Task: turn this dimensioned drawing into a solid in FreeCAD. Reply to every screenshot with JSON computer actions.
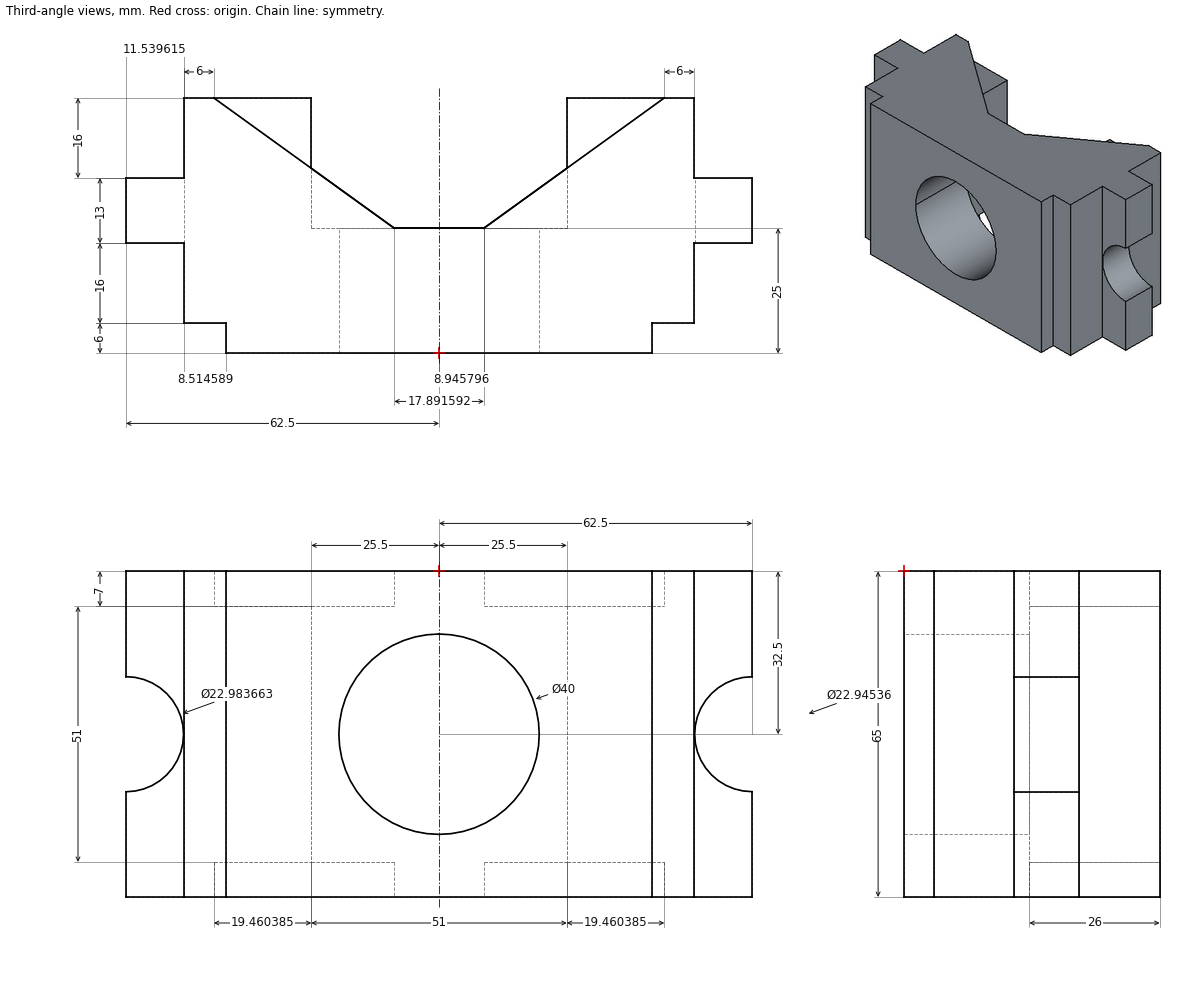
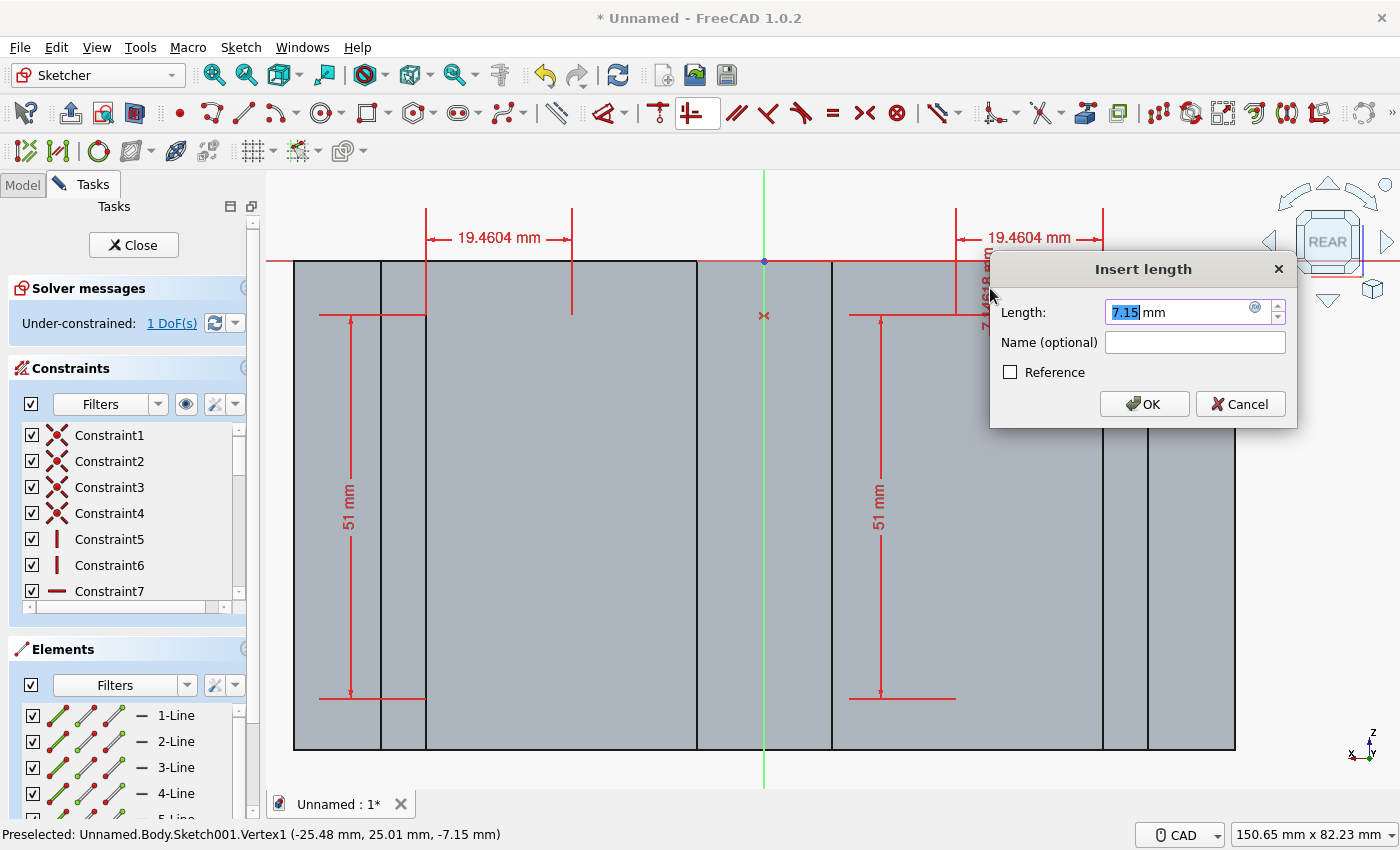
{"action": "type", "text": "7"}
{"action": "key", "text": "Return"}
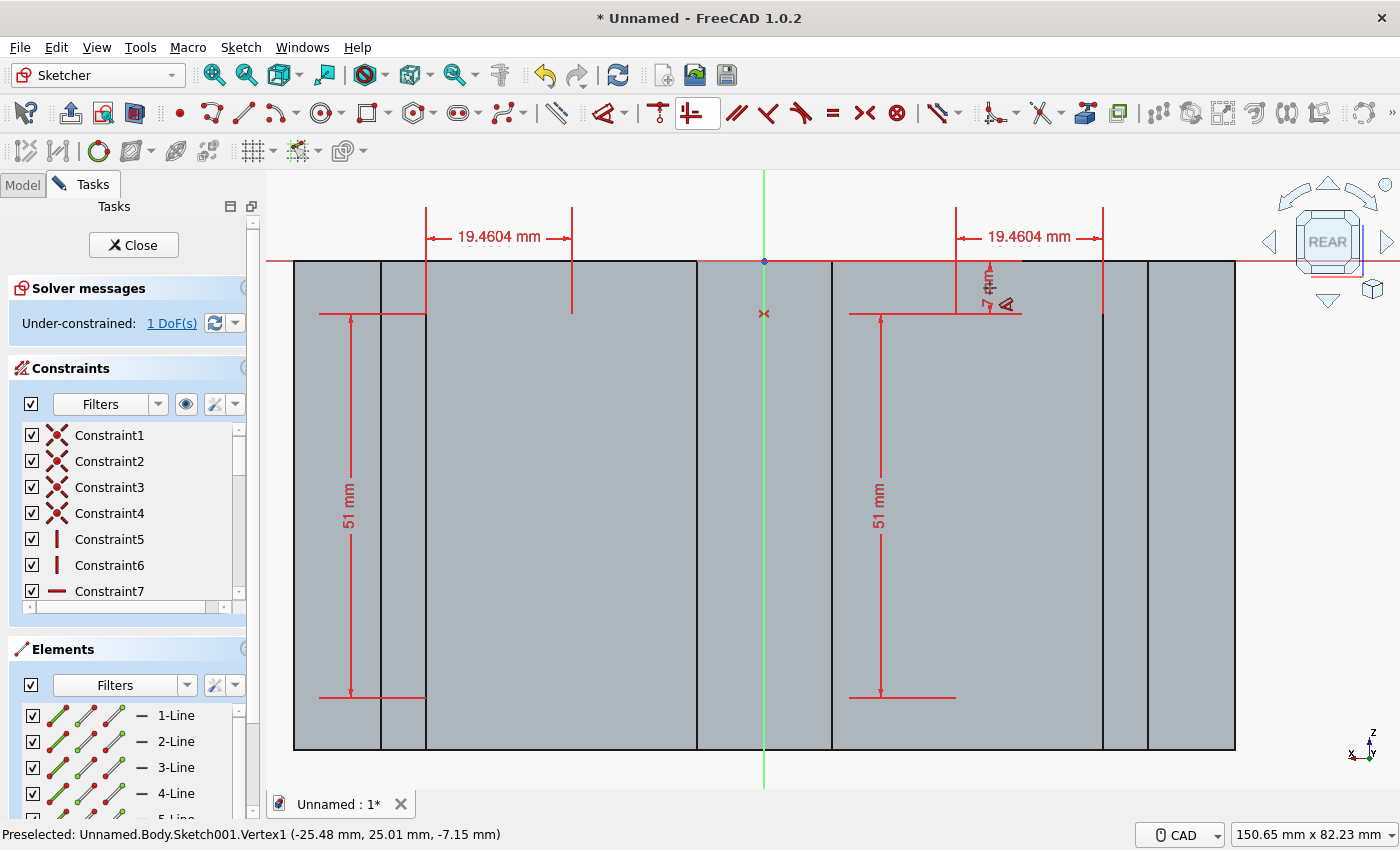
{"action": "left_click", "coordinate": [956, 314]}
{"action": "left_click", "coordinate": [860, 227]}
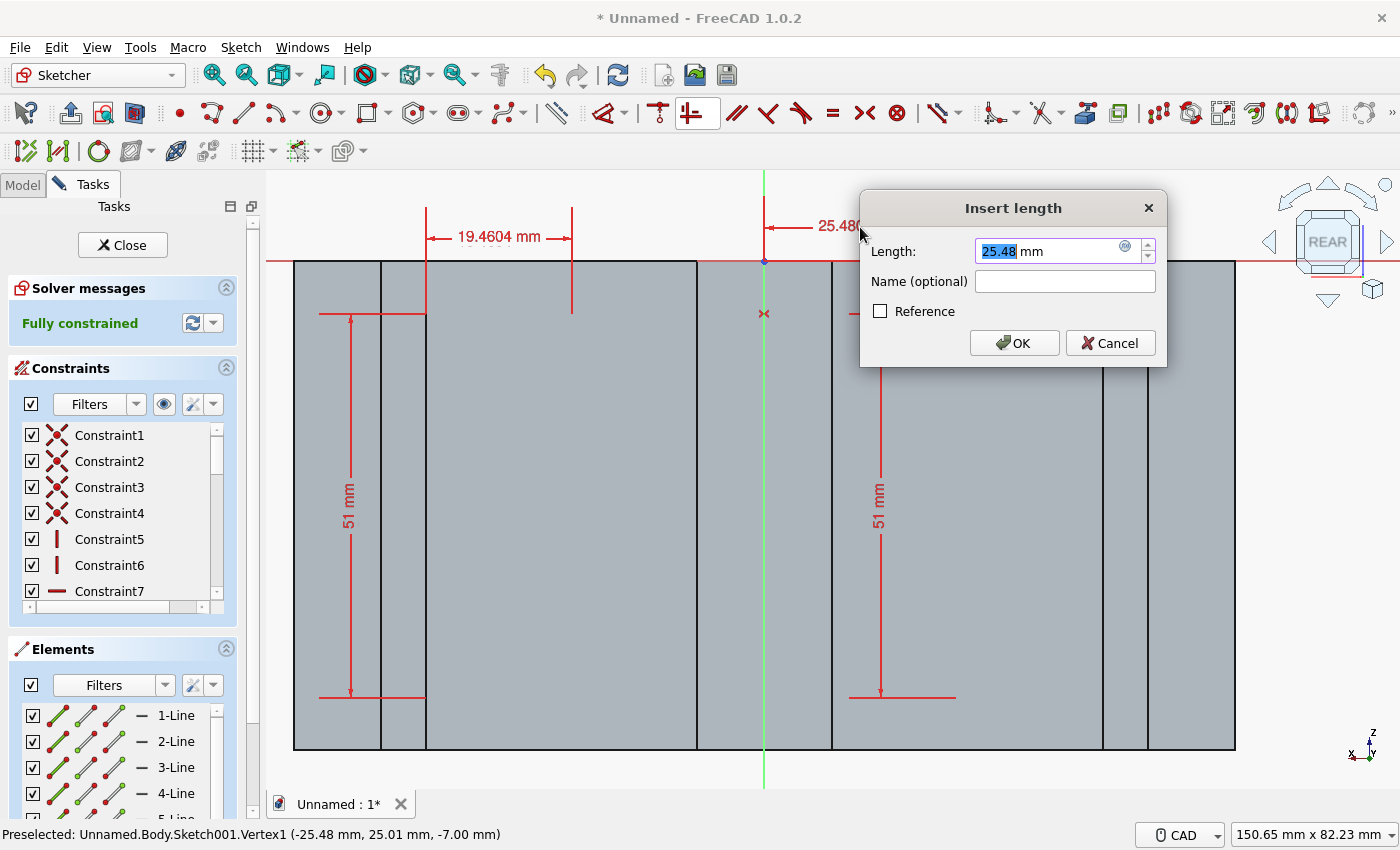
{"action": "type", "text": "25.5"}
{"action": "key", "text": "Return"}
{"action": "key", "text": "Escape"}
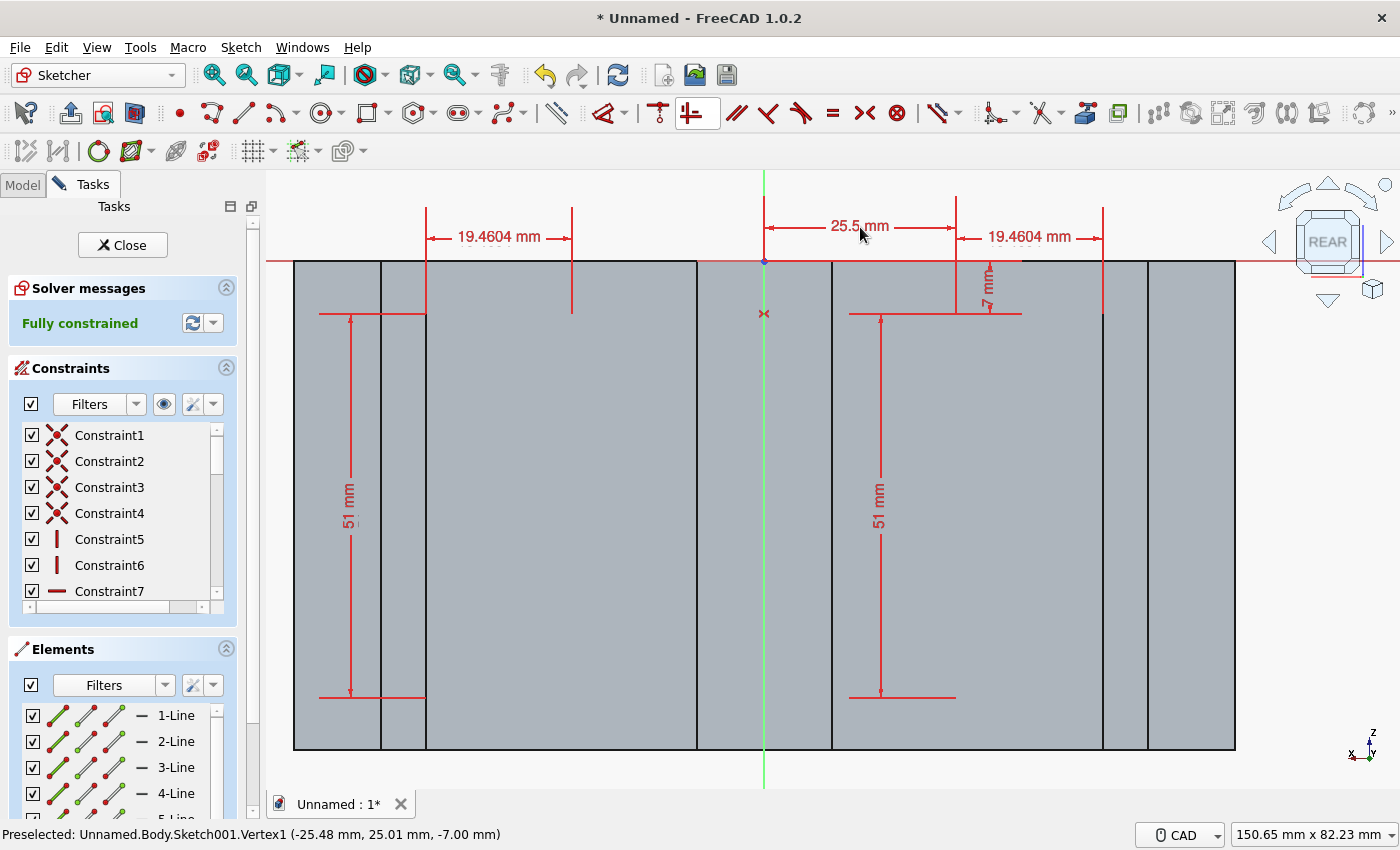
{"action": "left_click", "coordinate": [123, 245]}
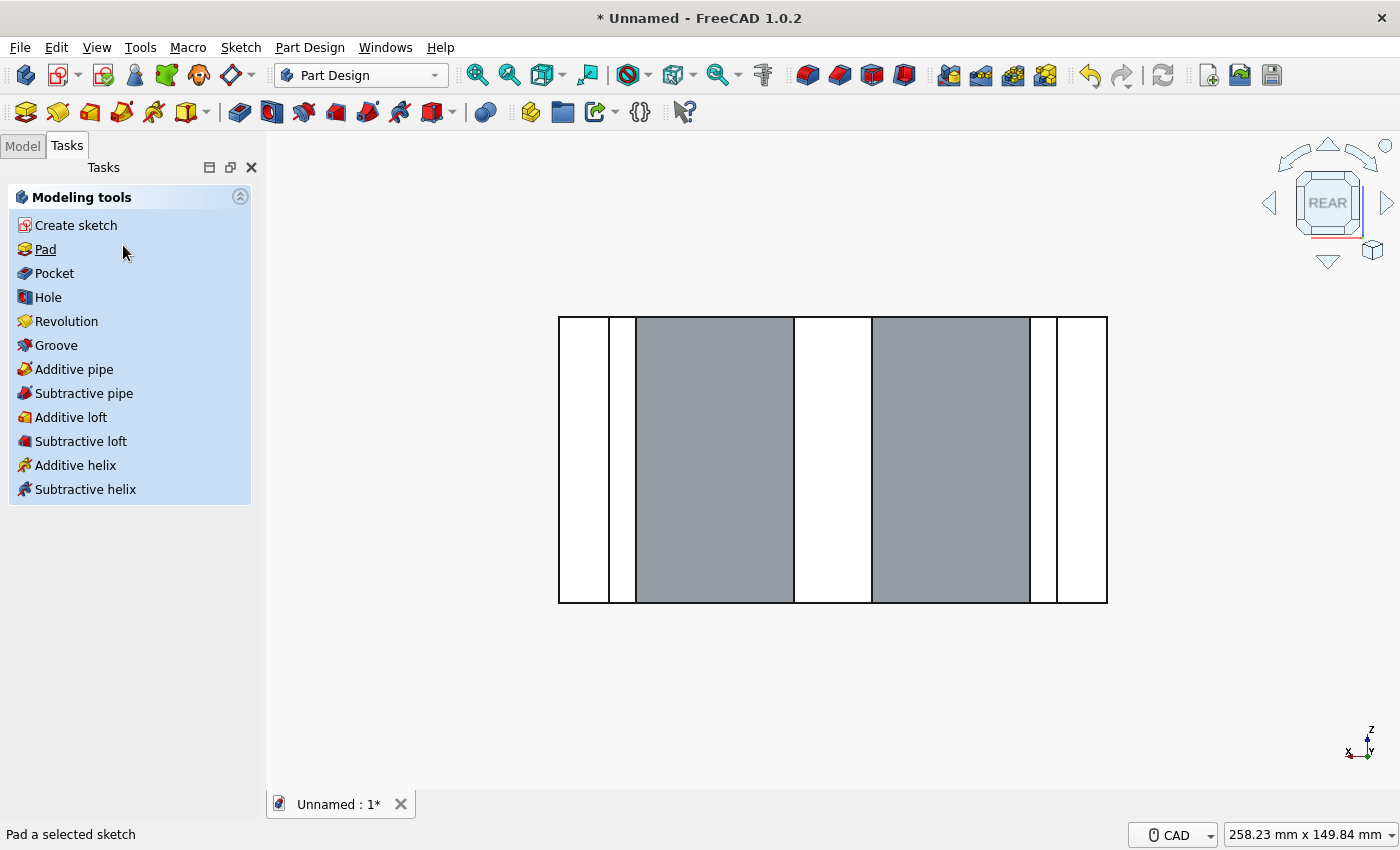
{"action": "left_click", "coordinate": [26, 112]}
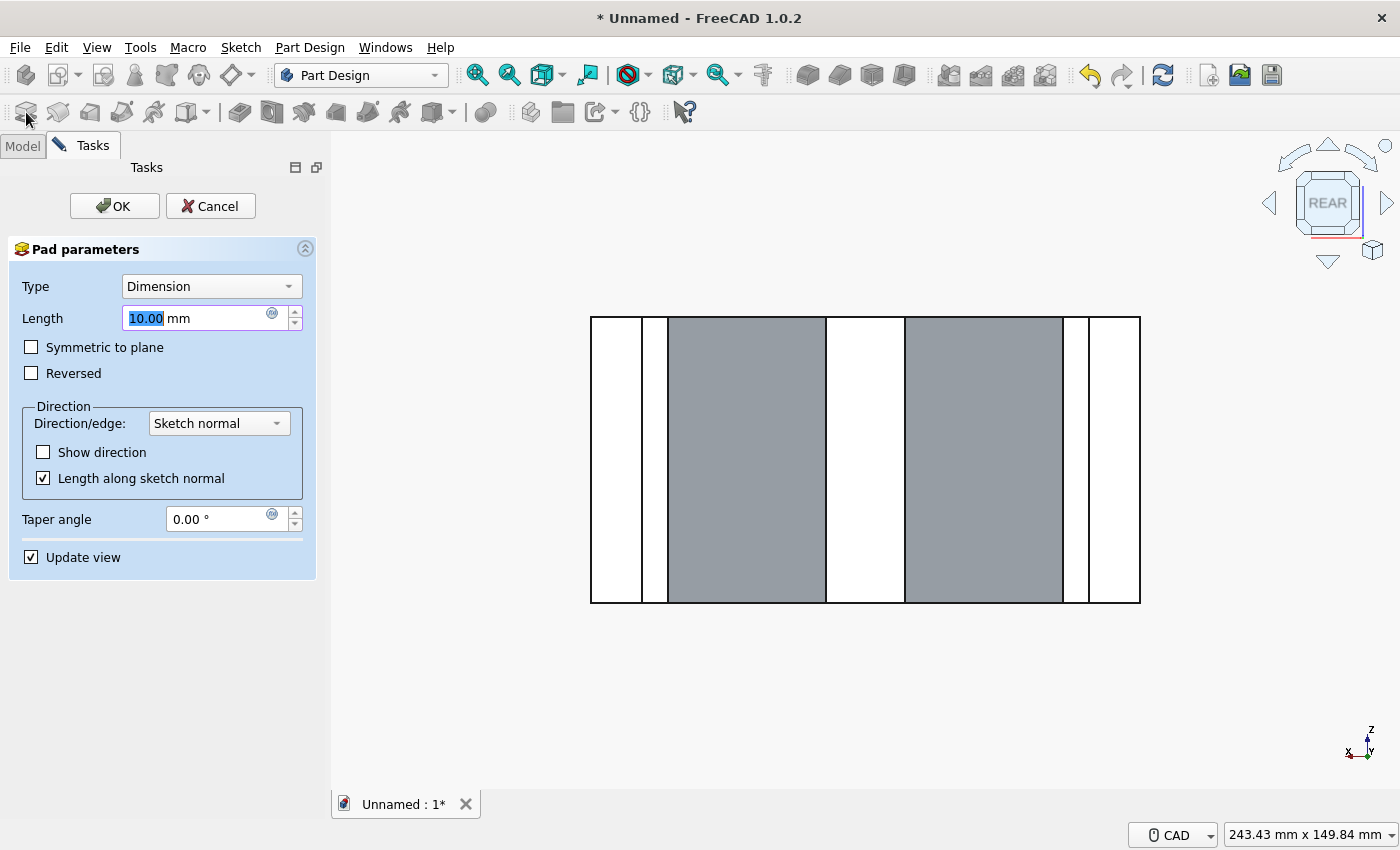
{"action": "type", "text": "26"}
{"action": "key", "text": "Tab"}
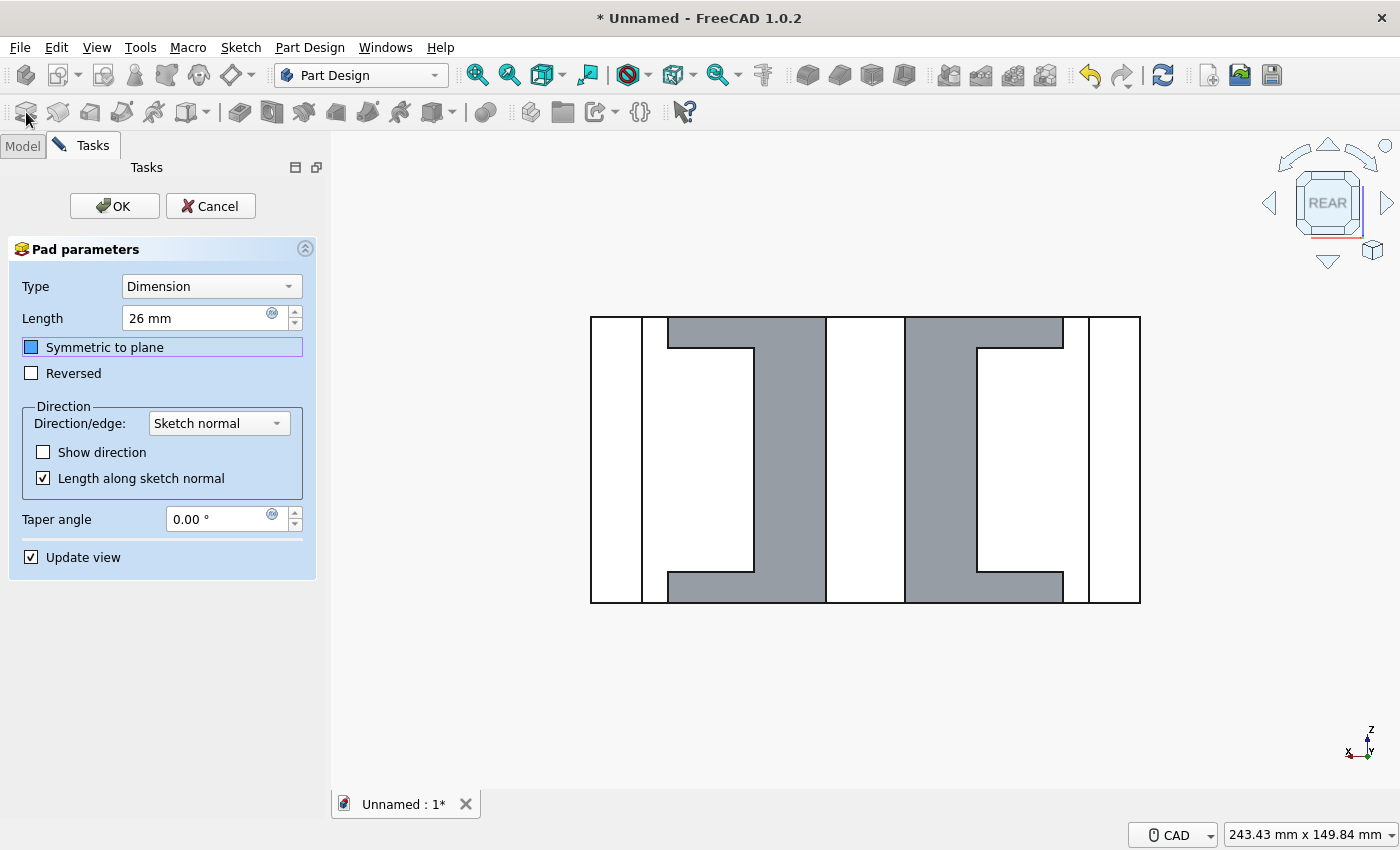
{"action": "left_click", "coordinate": [115, 206]}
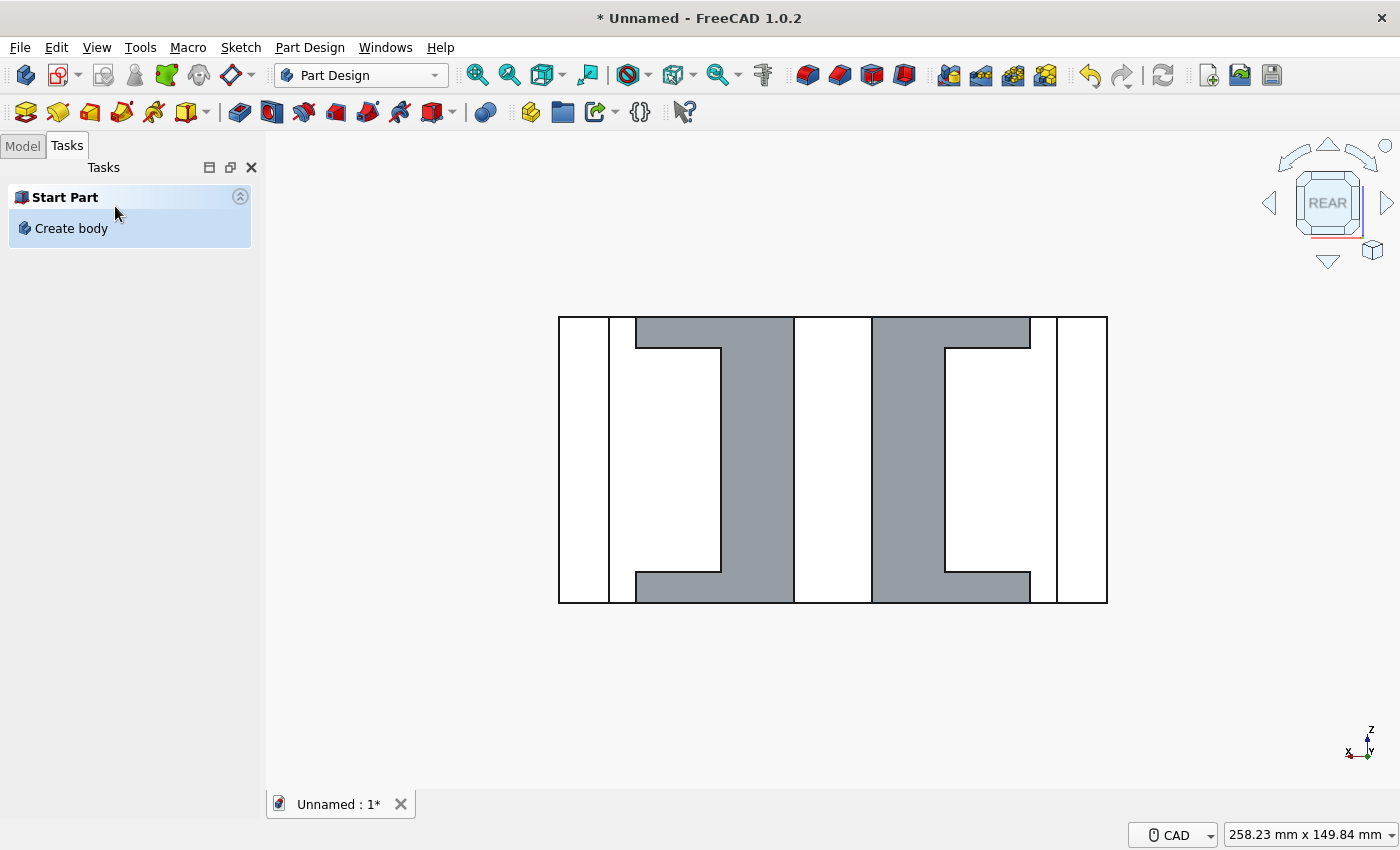
{"action": "left_click", "coordinate": [833, 377]}